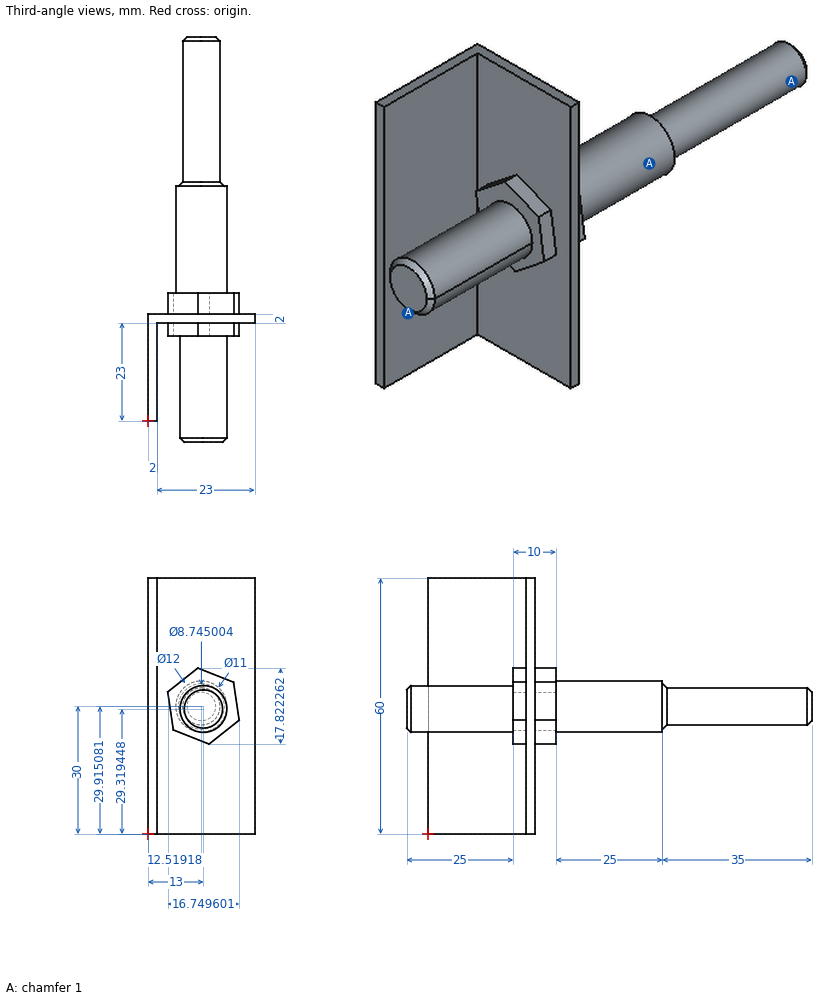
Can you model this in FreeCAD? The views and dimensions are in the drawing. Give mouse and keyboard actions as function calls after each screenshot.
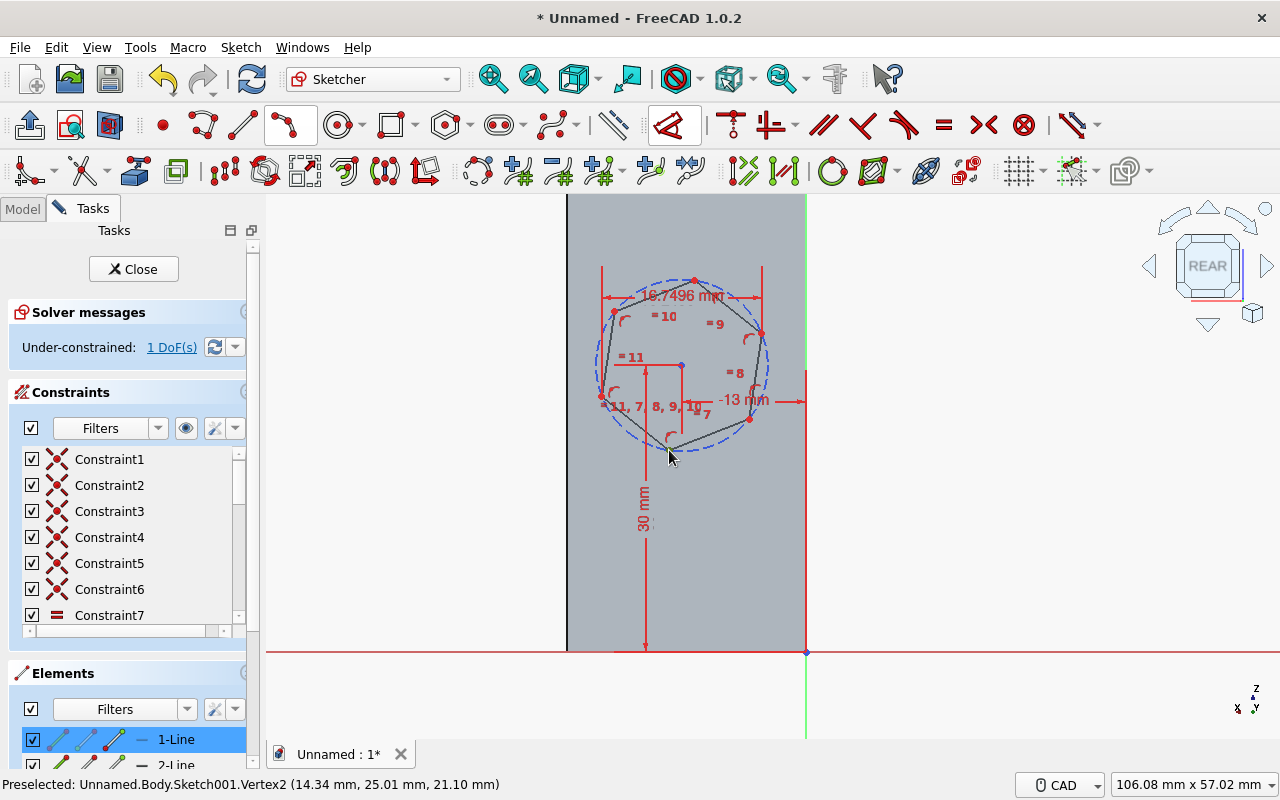
click(695, 280)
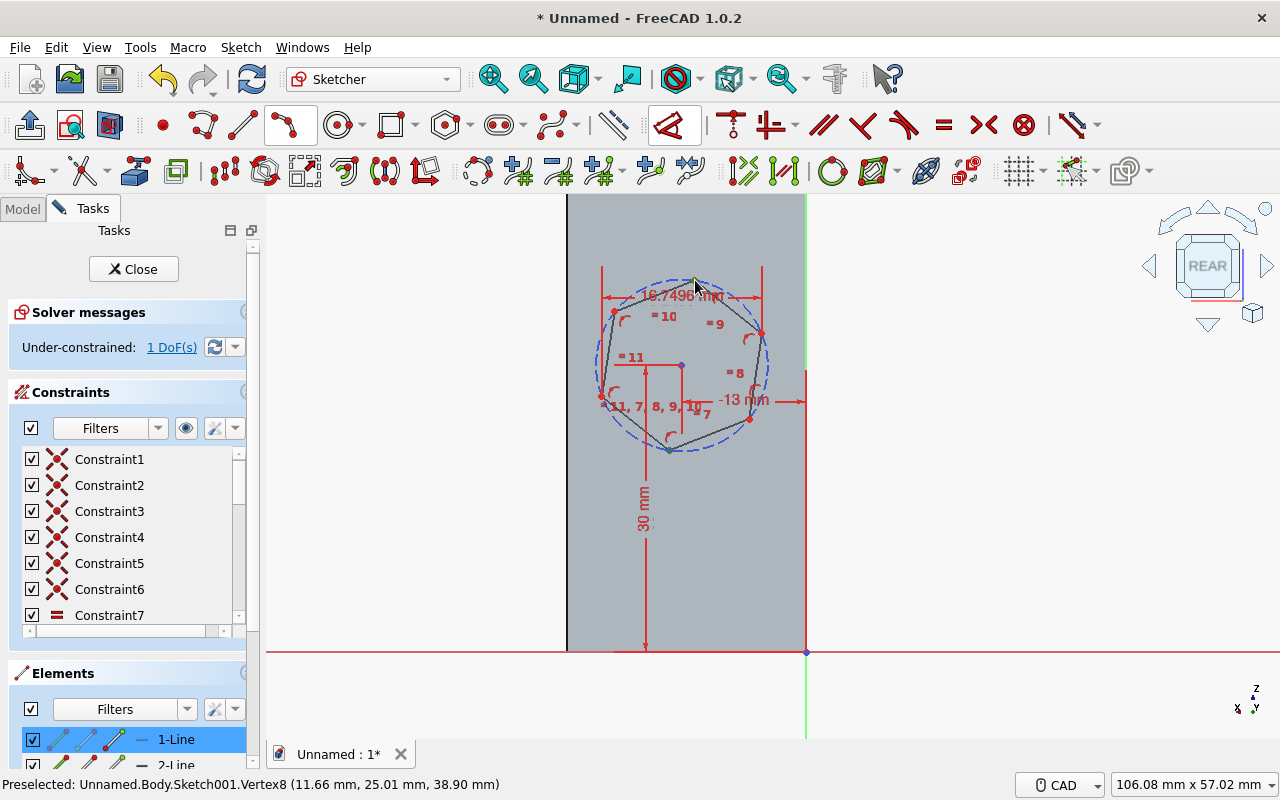
click(696, 126)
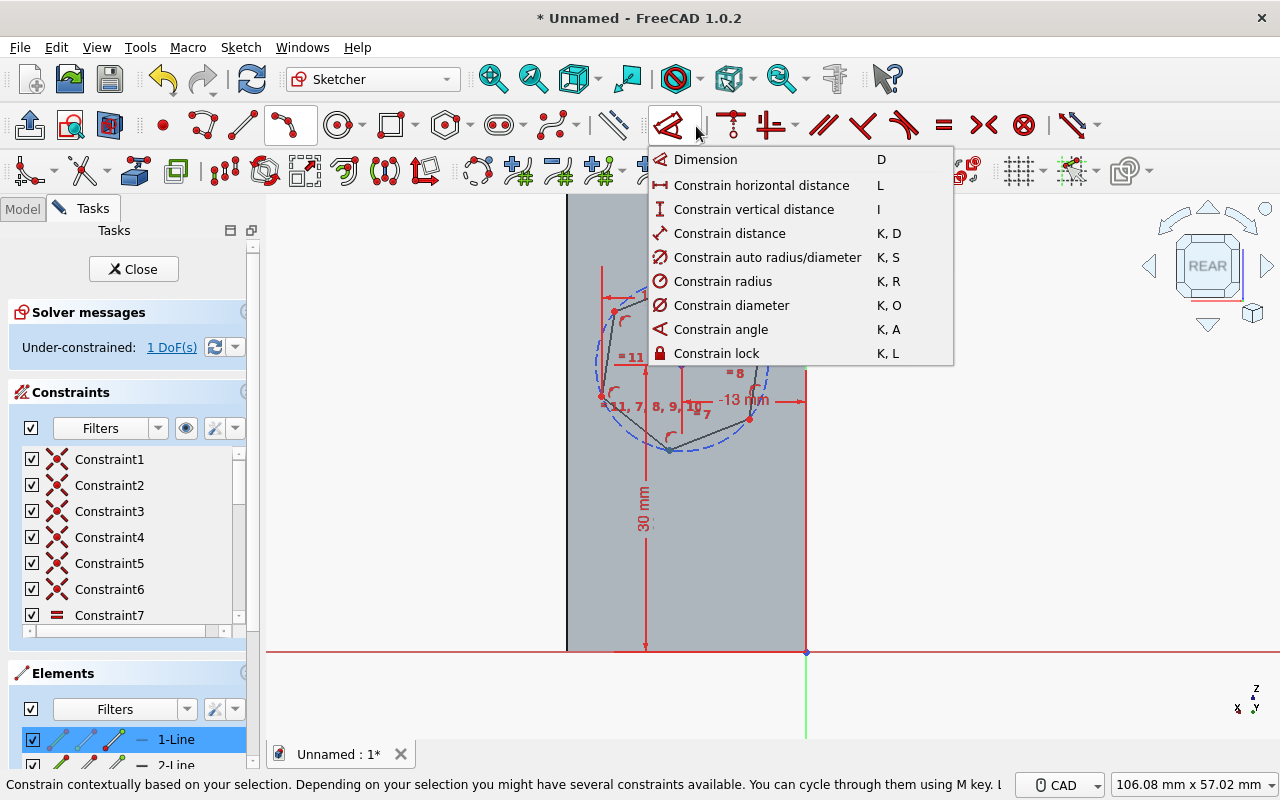
click(801, 209)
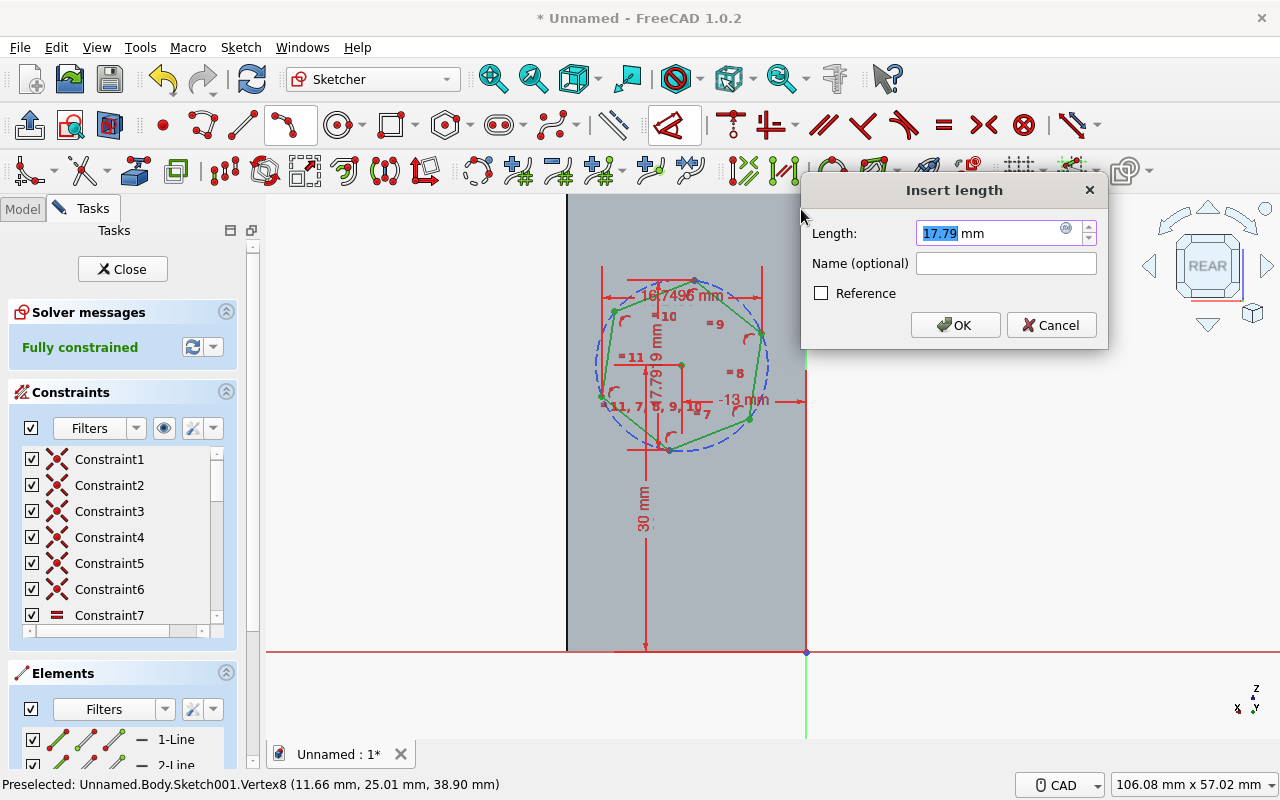
text(17.822262)
key(Return)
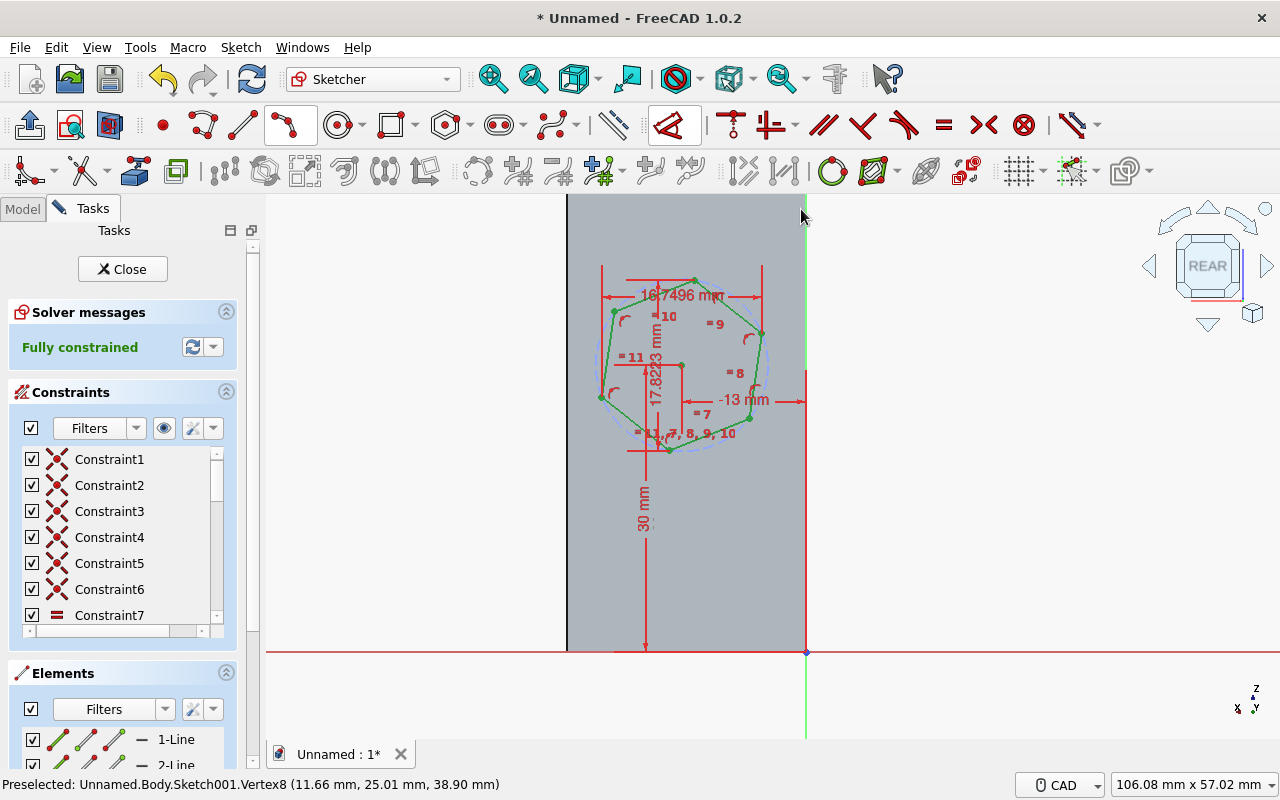
click(123, 269)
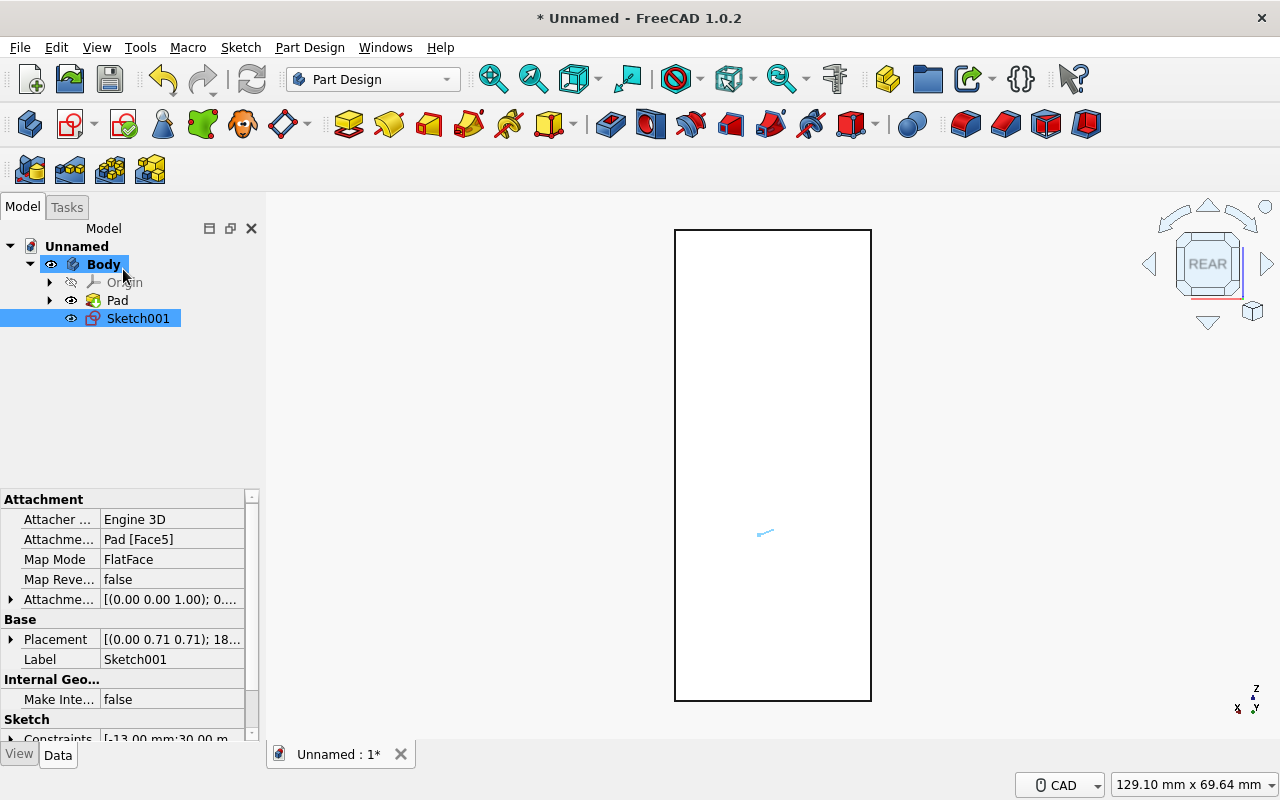
click(350, 124)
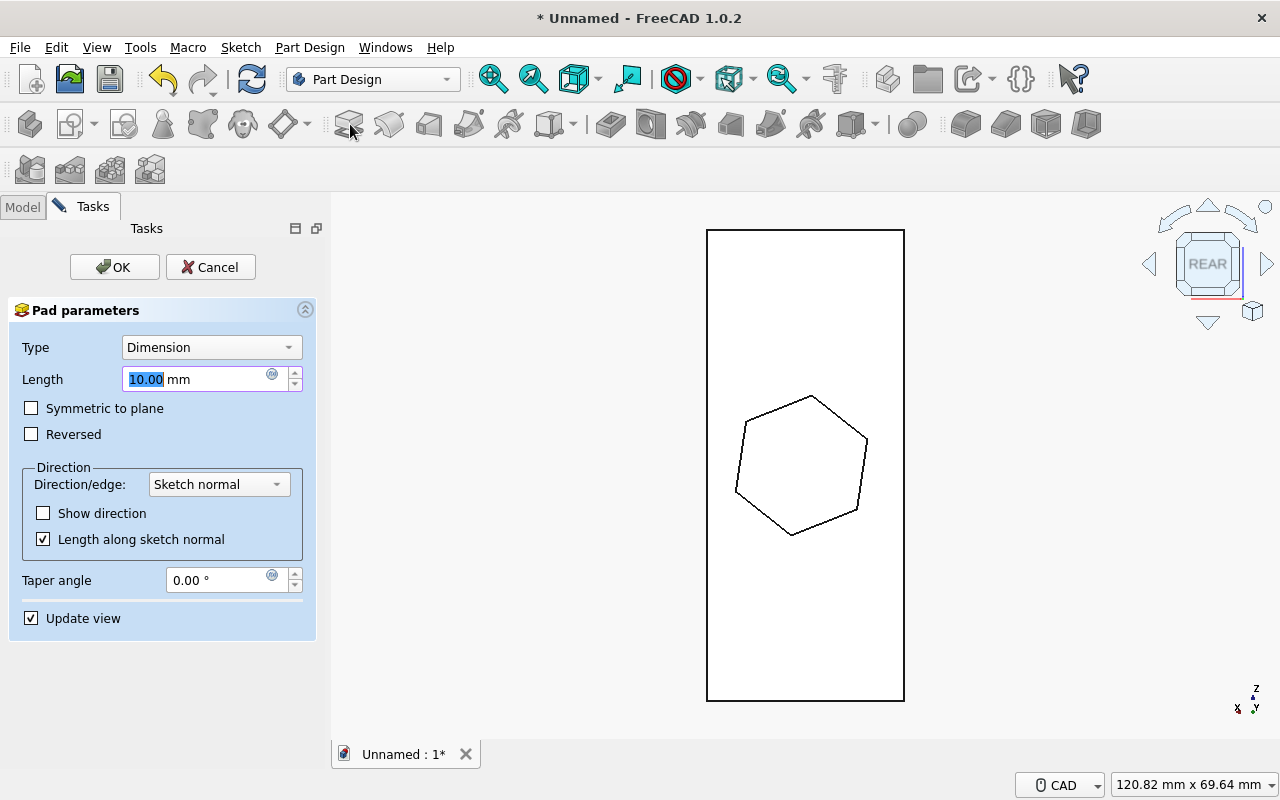
text(10)
key(Tab)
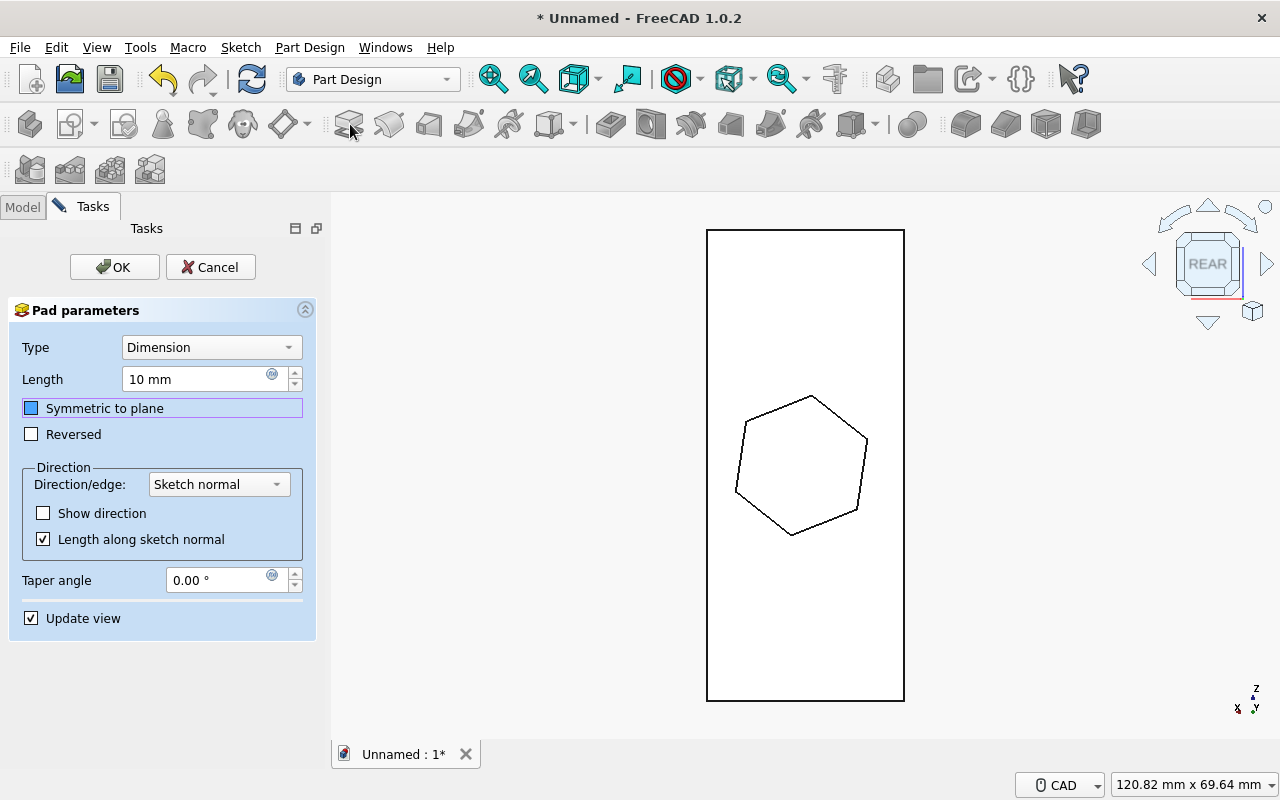
click(30, 408)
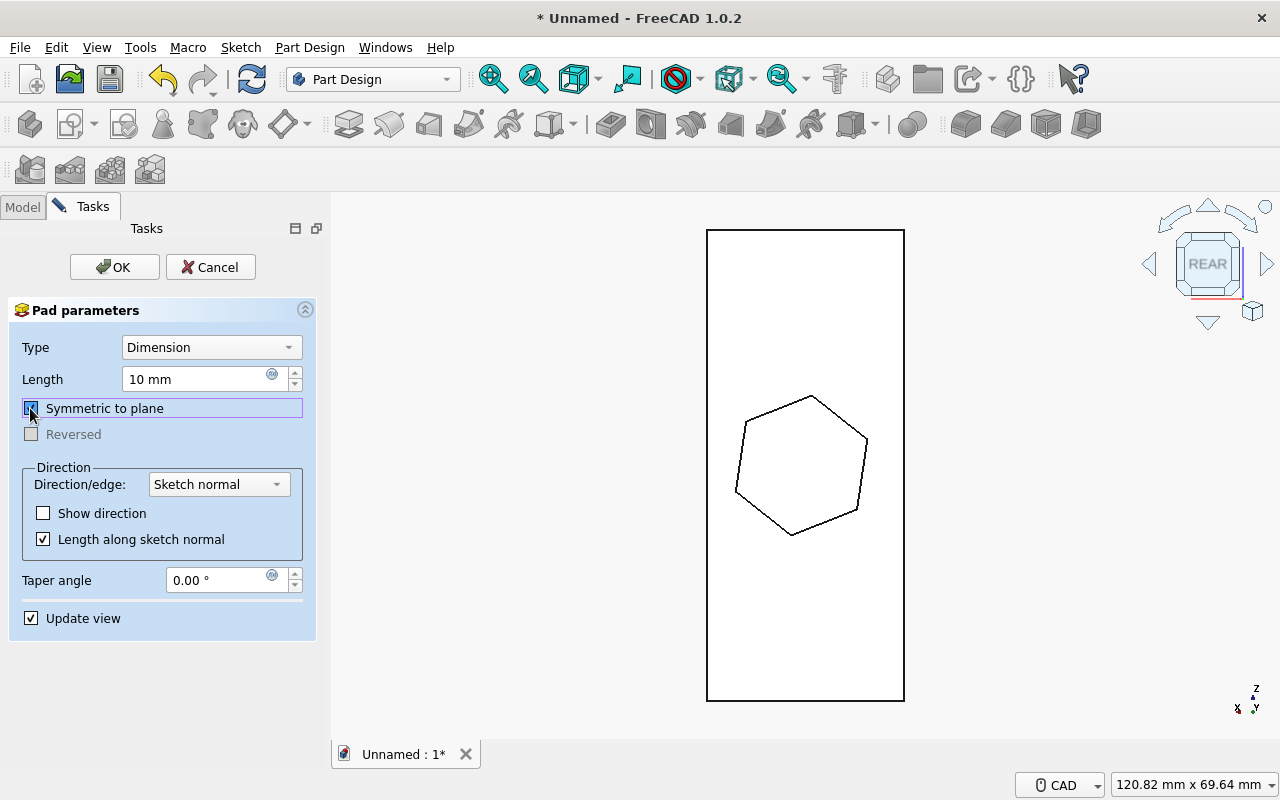
click(115, 267)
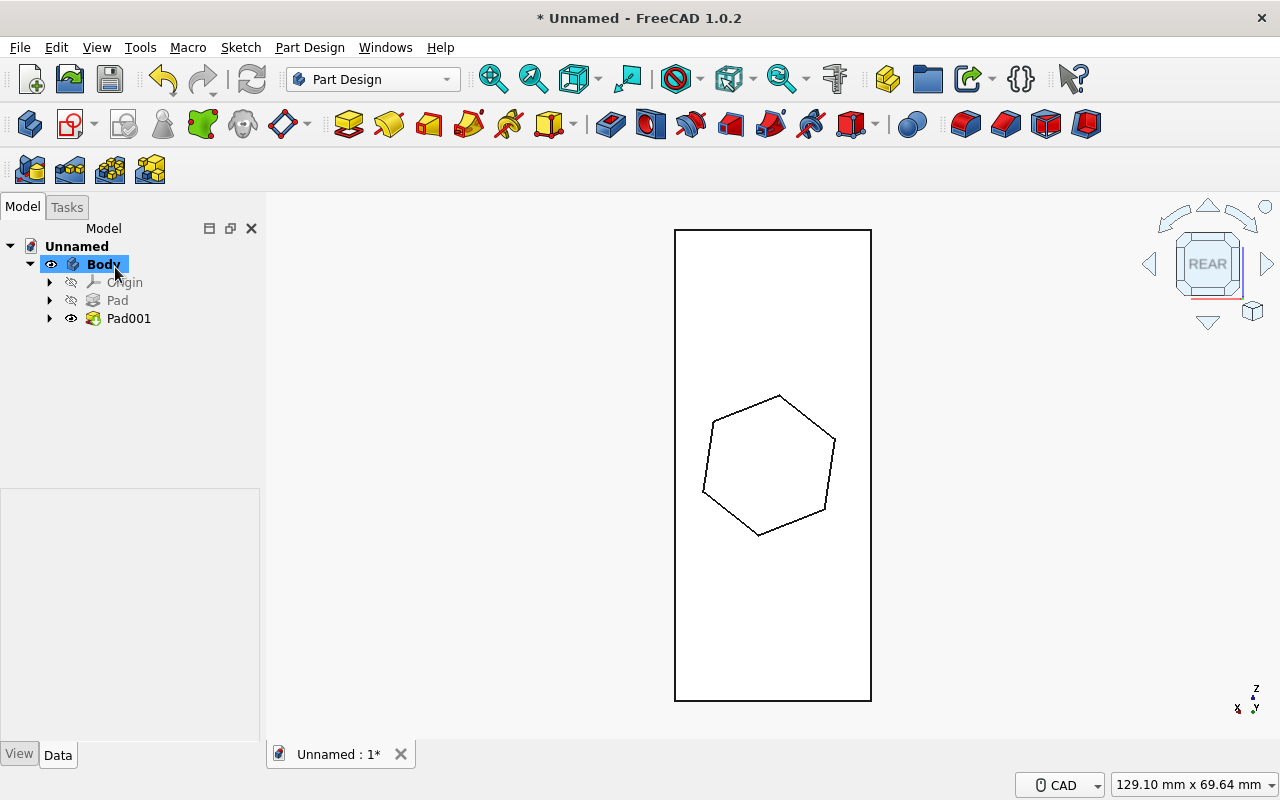
key(0)